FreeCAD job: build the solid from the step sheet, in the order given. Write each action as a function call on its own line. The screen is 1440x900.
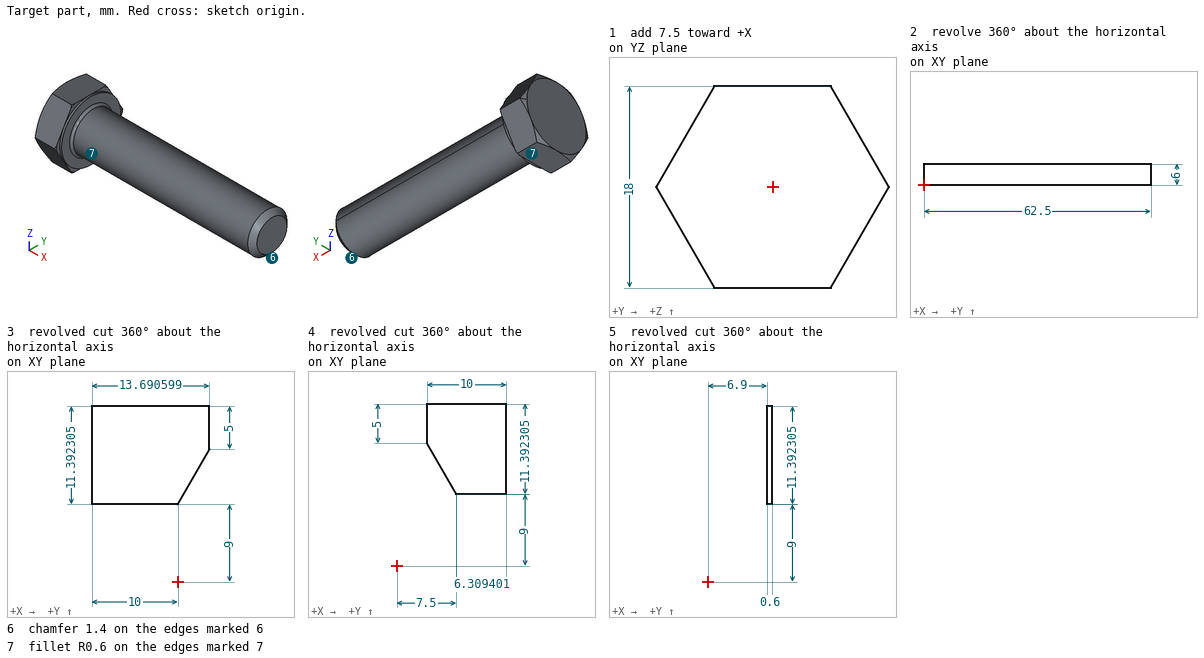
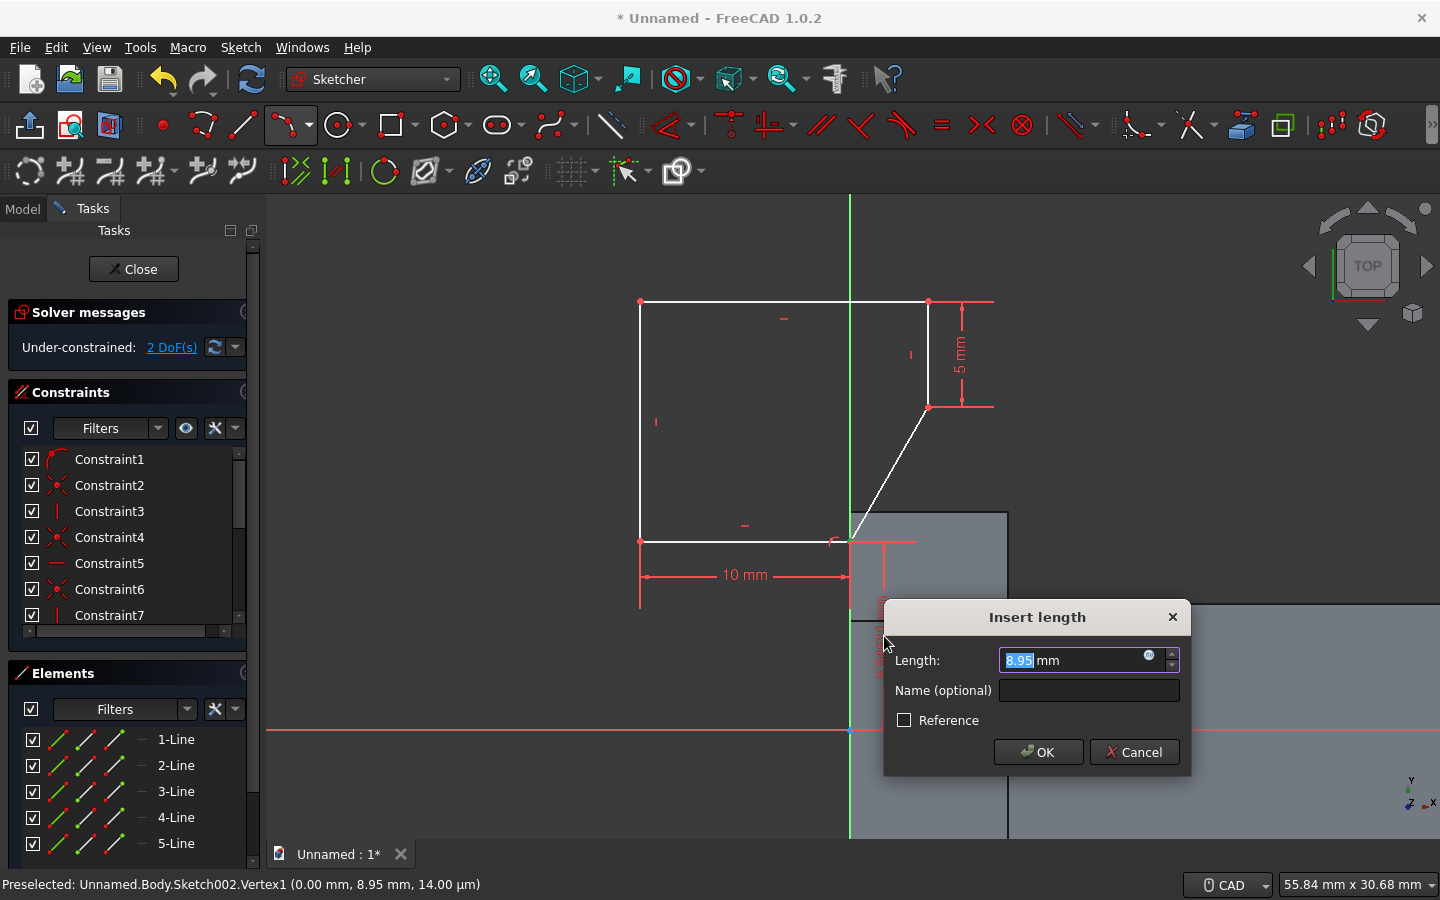
text(9)
key(Return)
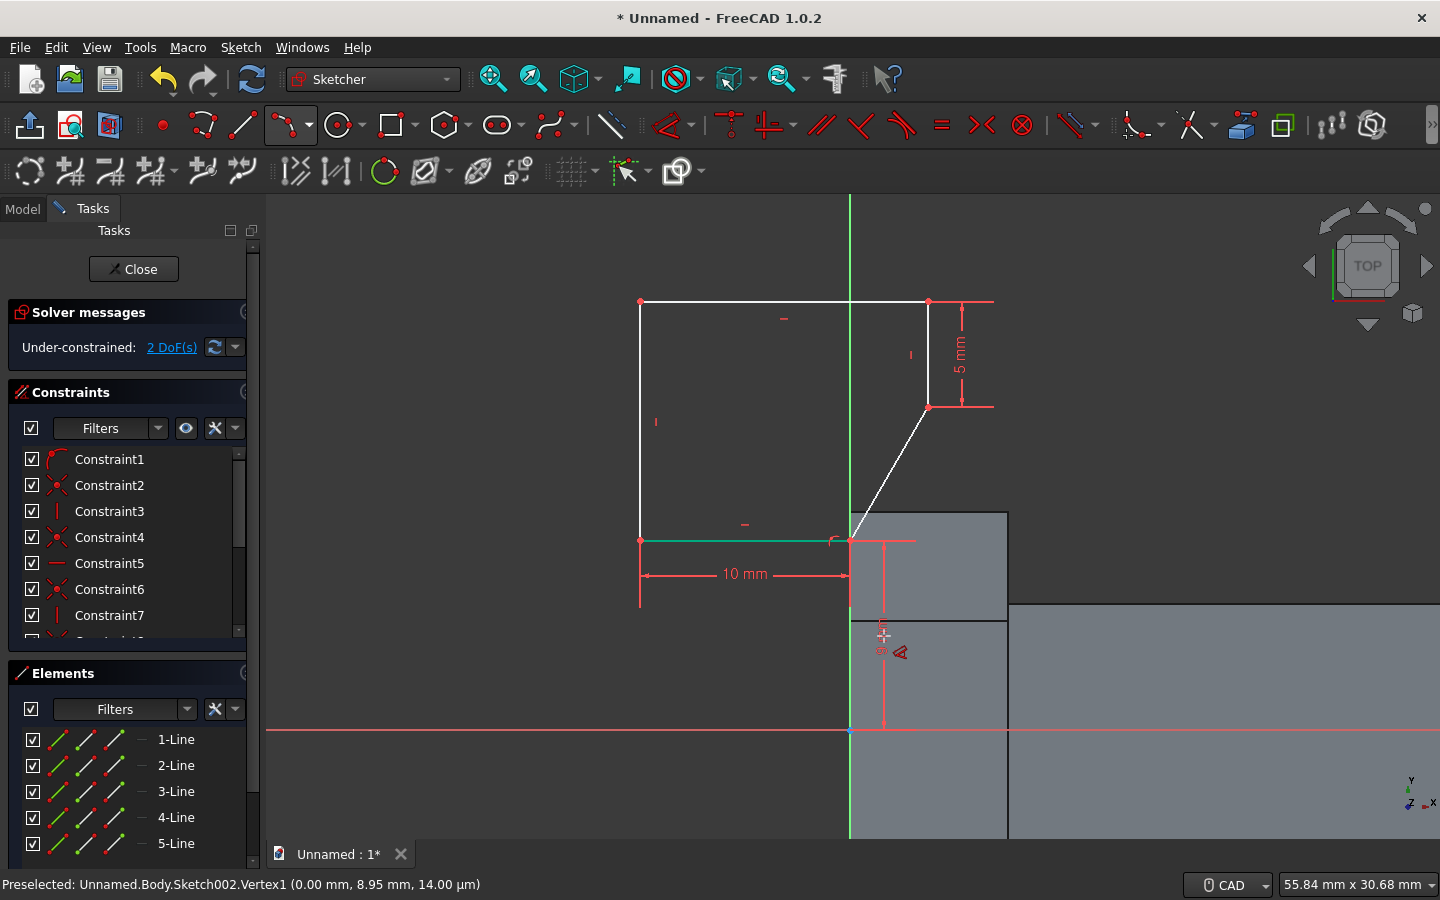
click(727, 302)
click(784, 268)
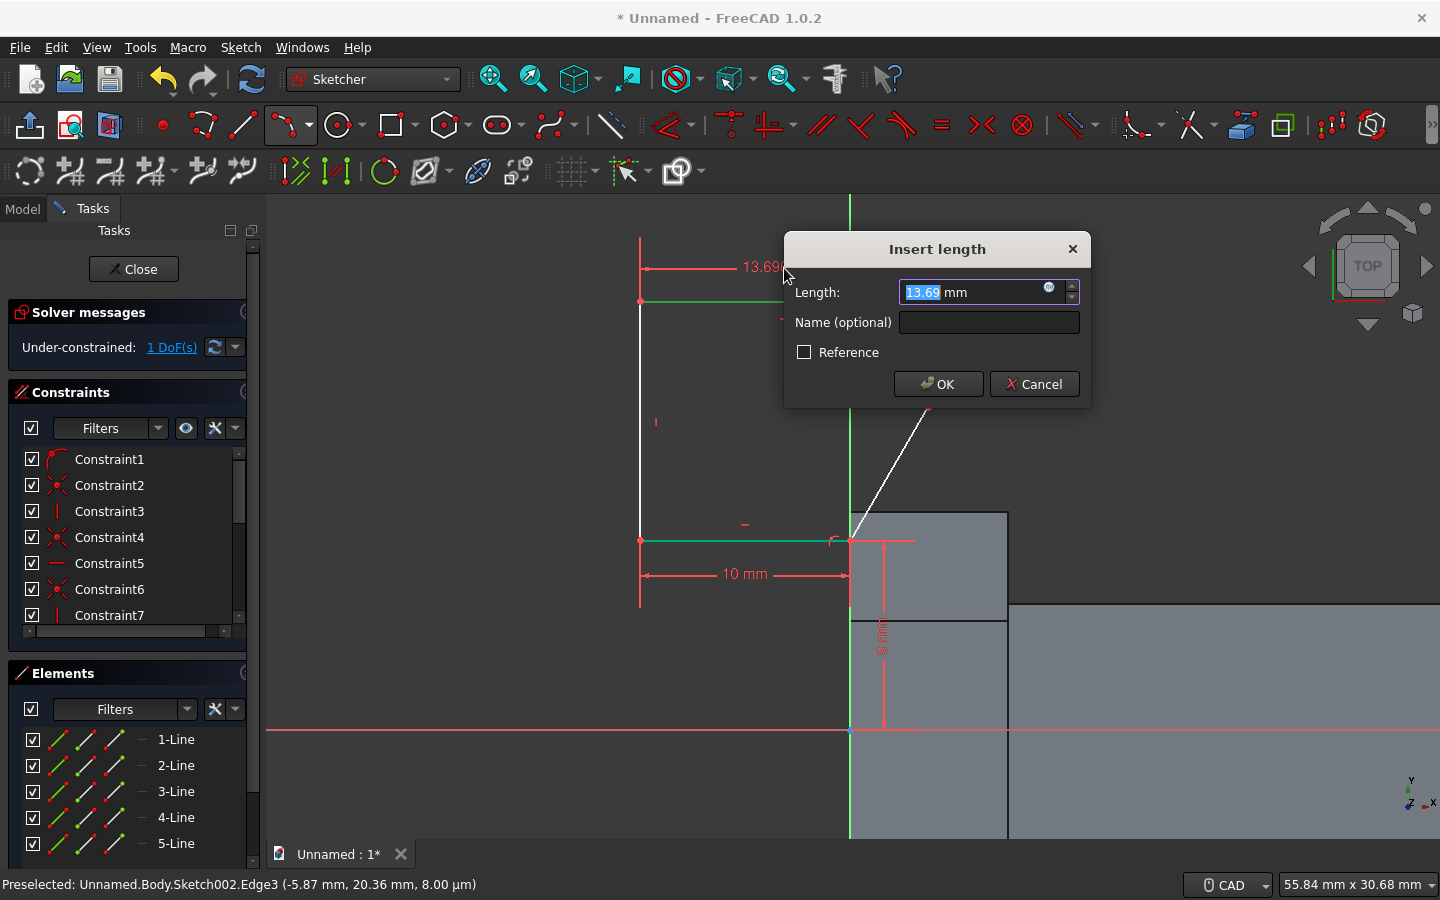
text(13.690599)
key(Return)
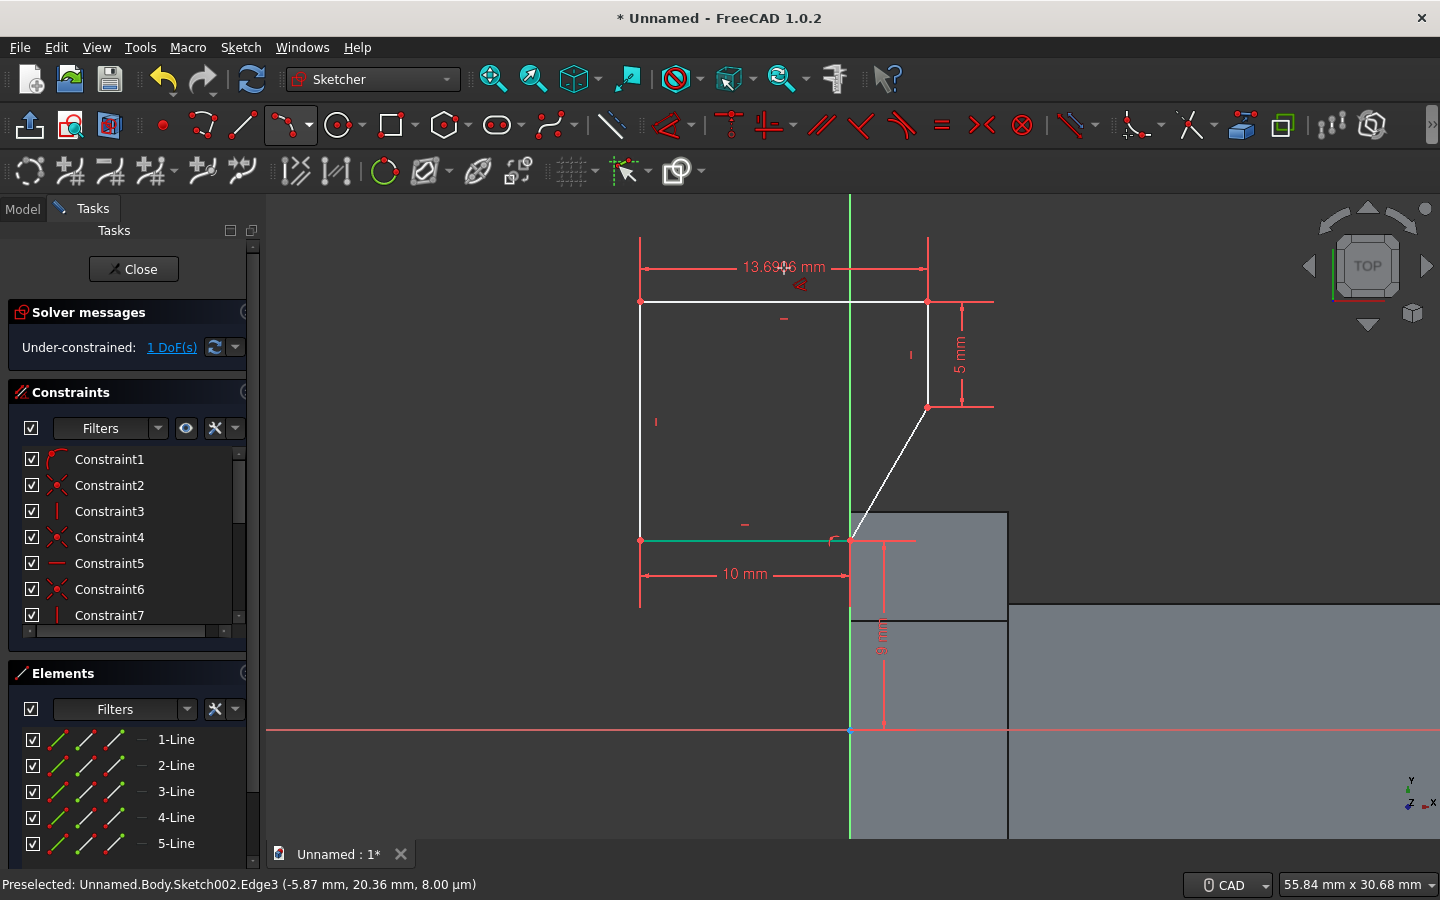
click(640, 374)
click(606, 421)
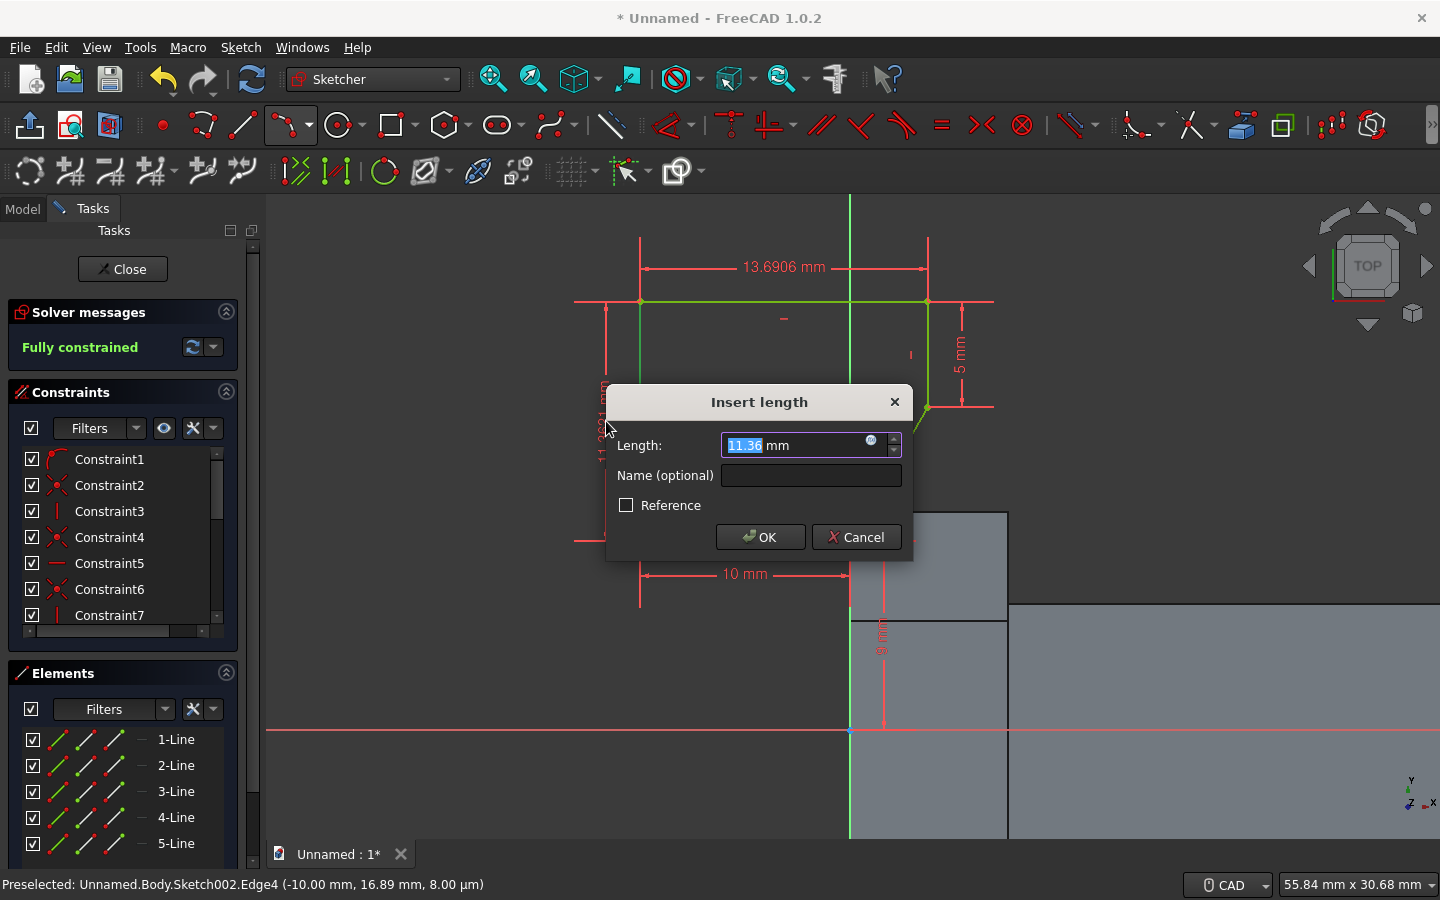
text(11.392305)
key(Return)
key(Escape)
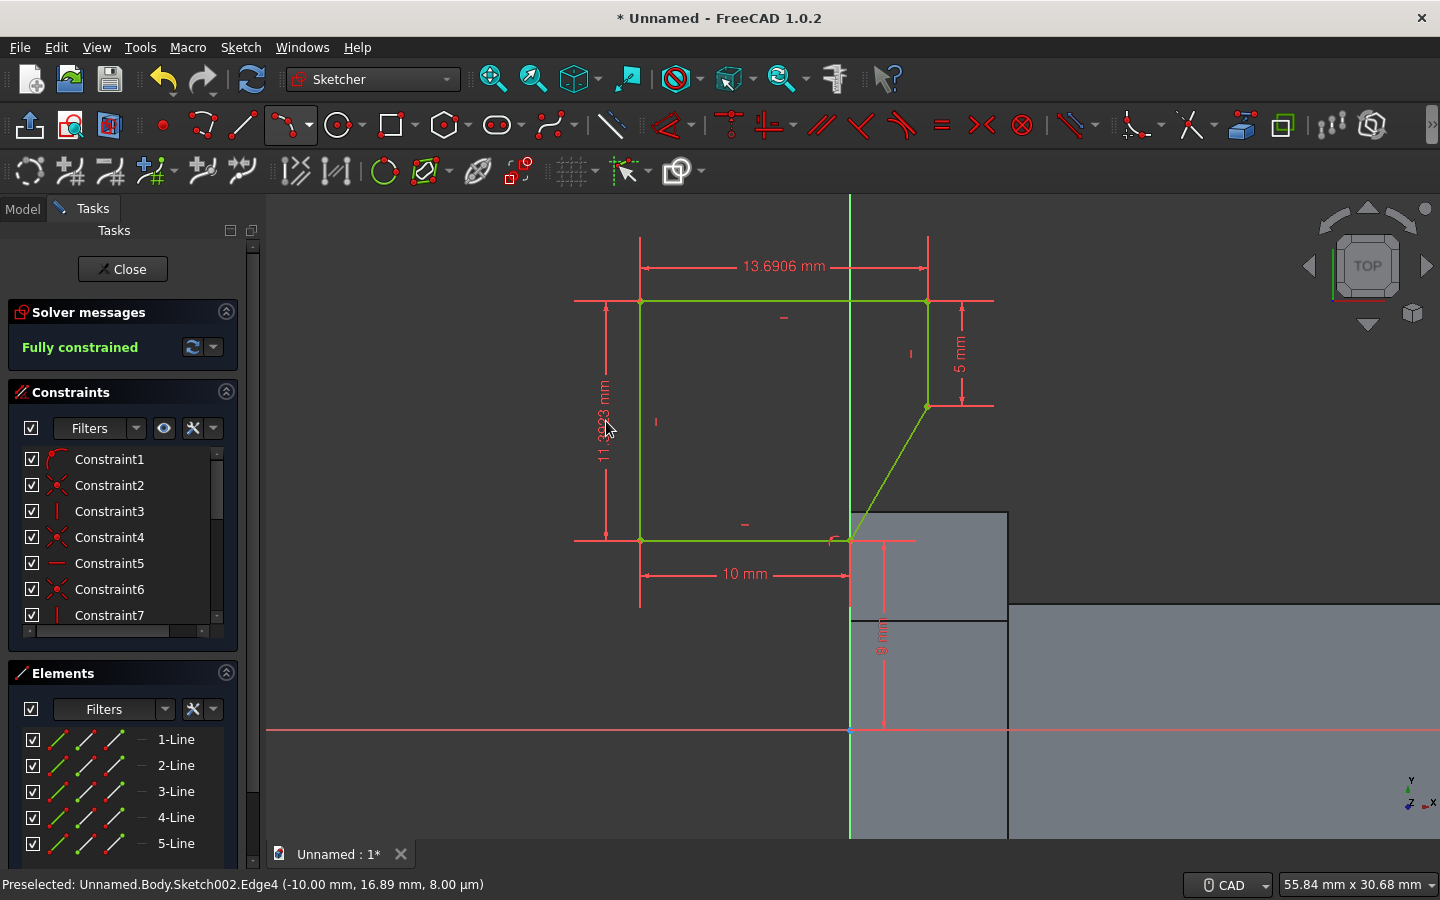
click(123, 269)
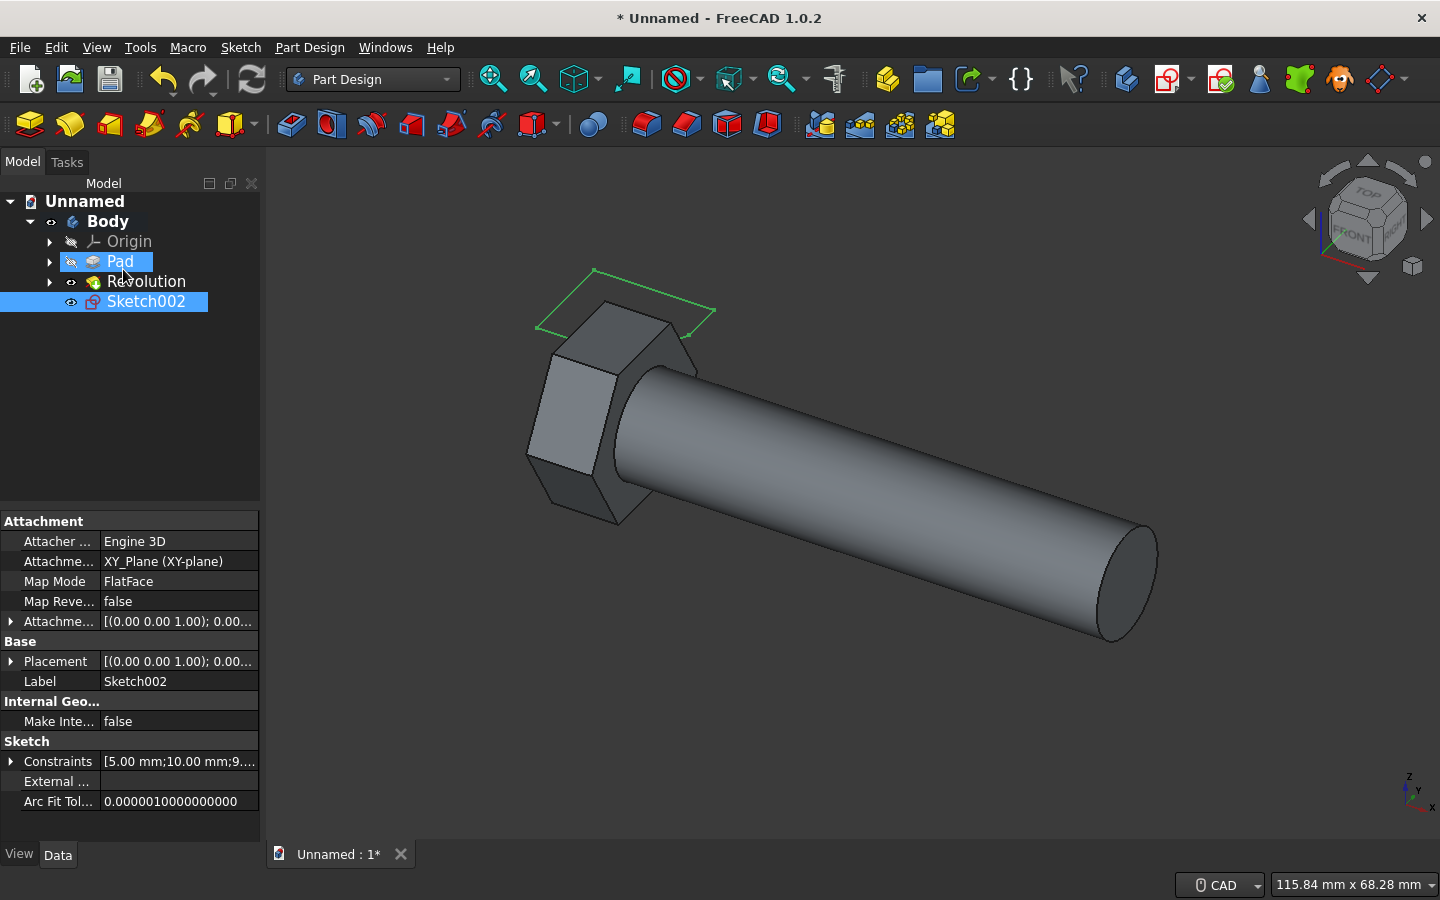
click(372, 124)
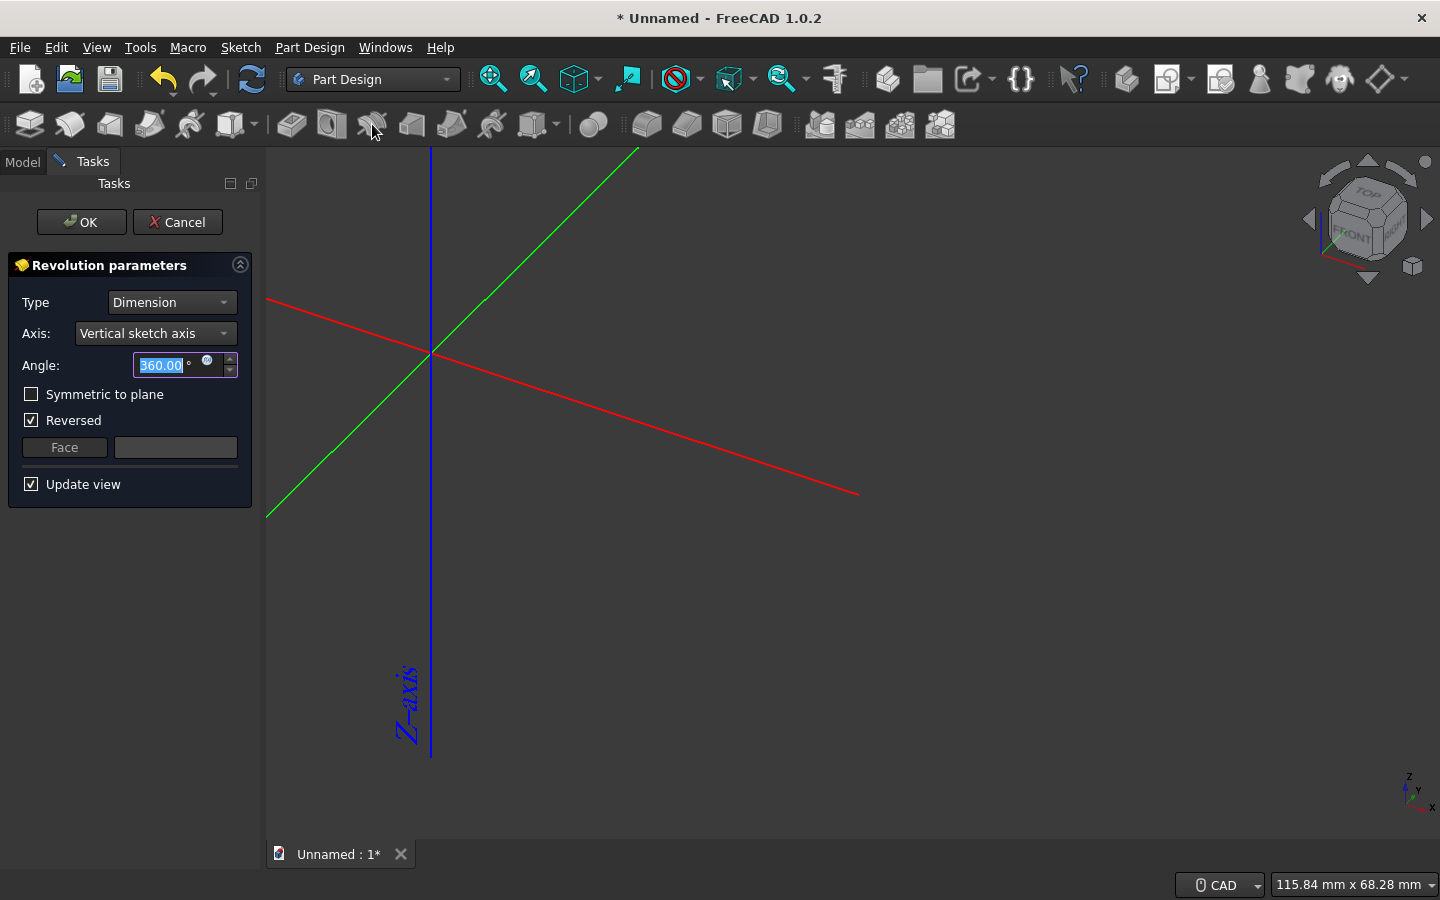
click(156, 334)